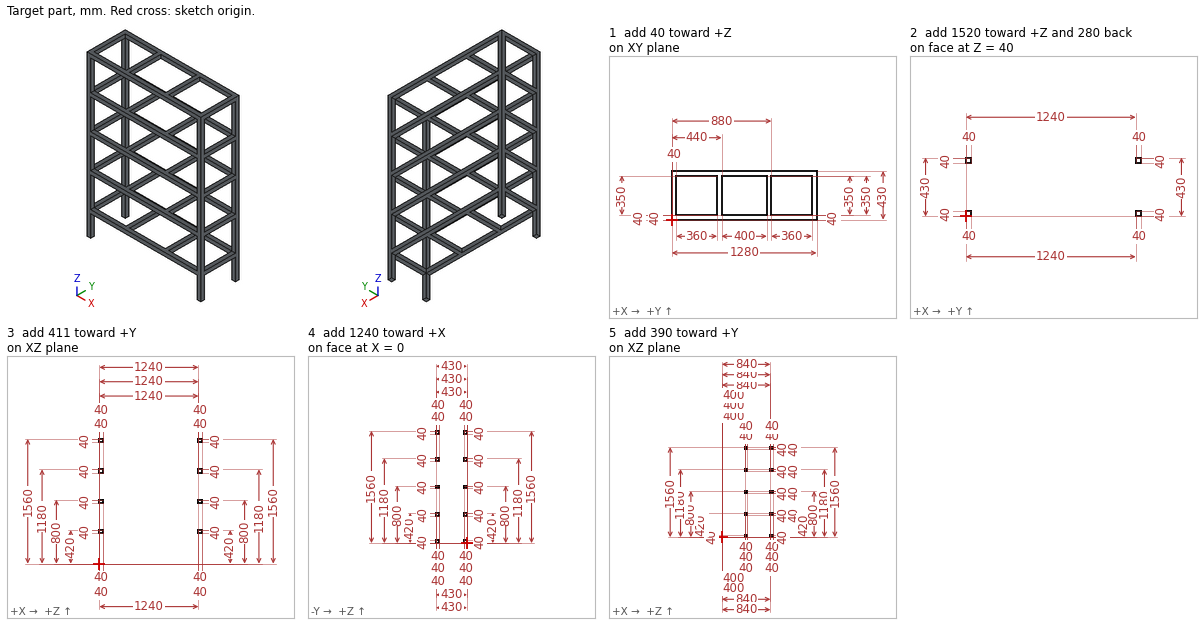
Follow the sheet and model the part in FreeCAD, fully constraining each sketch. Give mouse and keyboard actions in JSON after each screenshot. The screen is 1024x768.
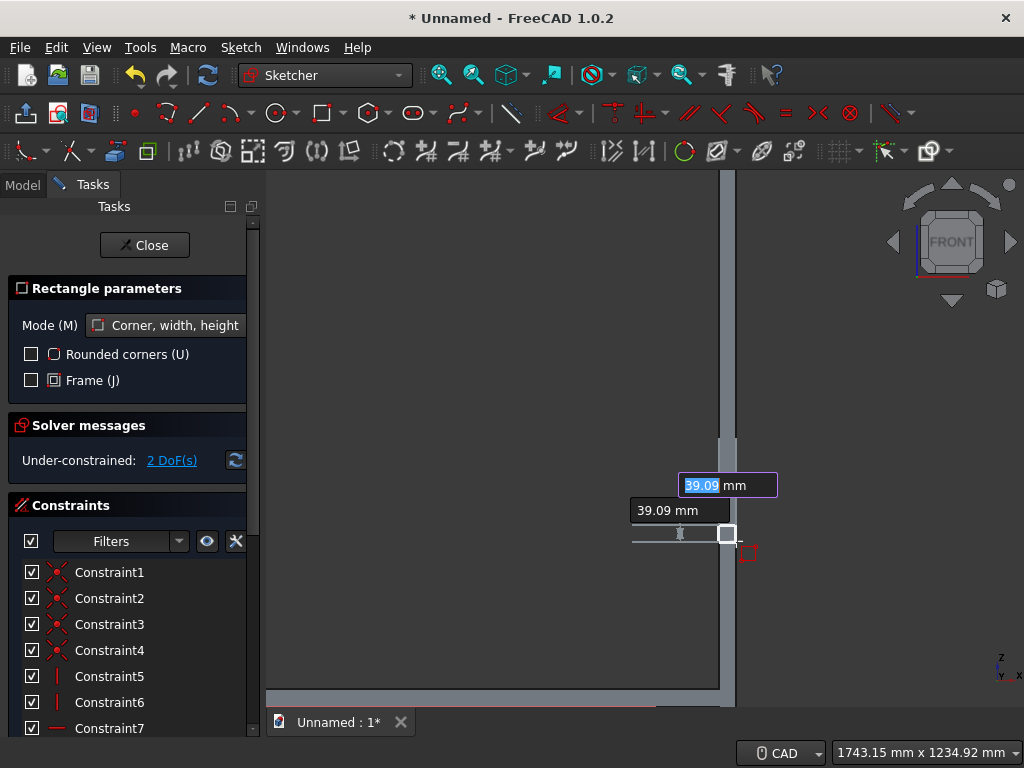
{"action": "type", "text": "40"}
{"action": "key", "text": "Tab"}
{"action": "type", "text": "40"}
{"action": "key", "text": "Return"}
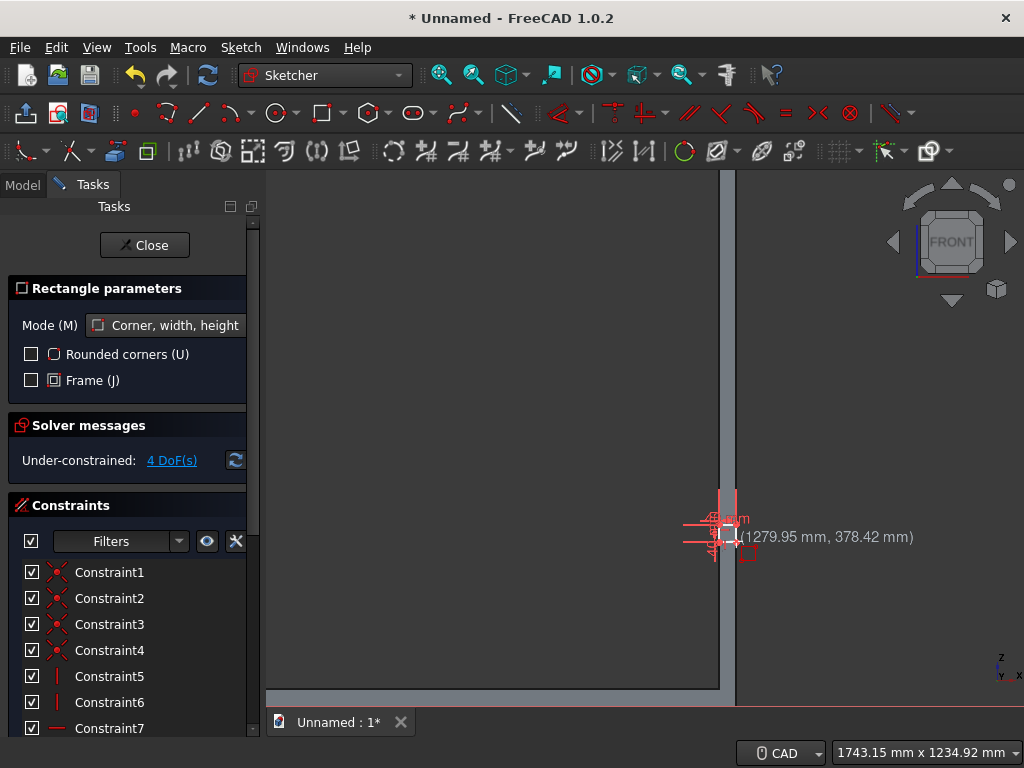
{"action": "scroll", "coordinate": [721, 525], "scroll_direction": "down", "scroll_amount": 3}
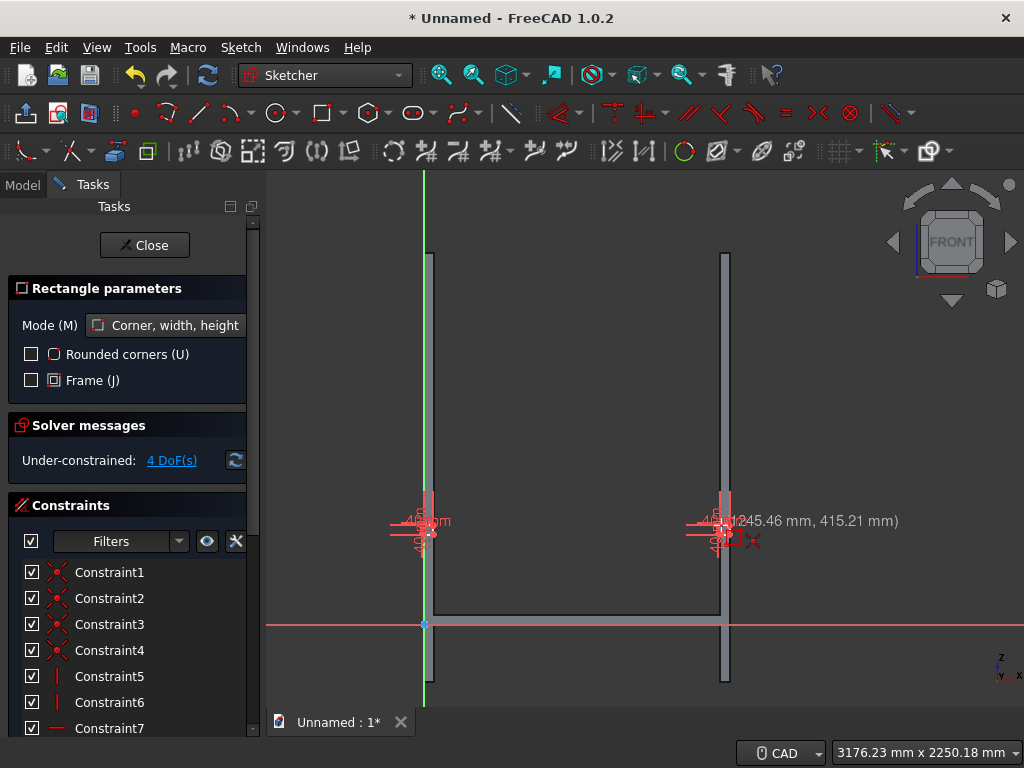
{"action": "scroll", "coordinate": [424, 434], "scroll_direction": "up", "scroll_amount": 3}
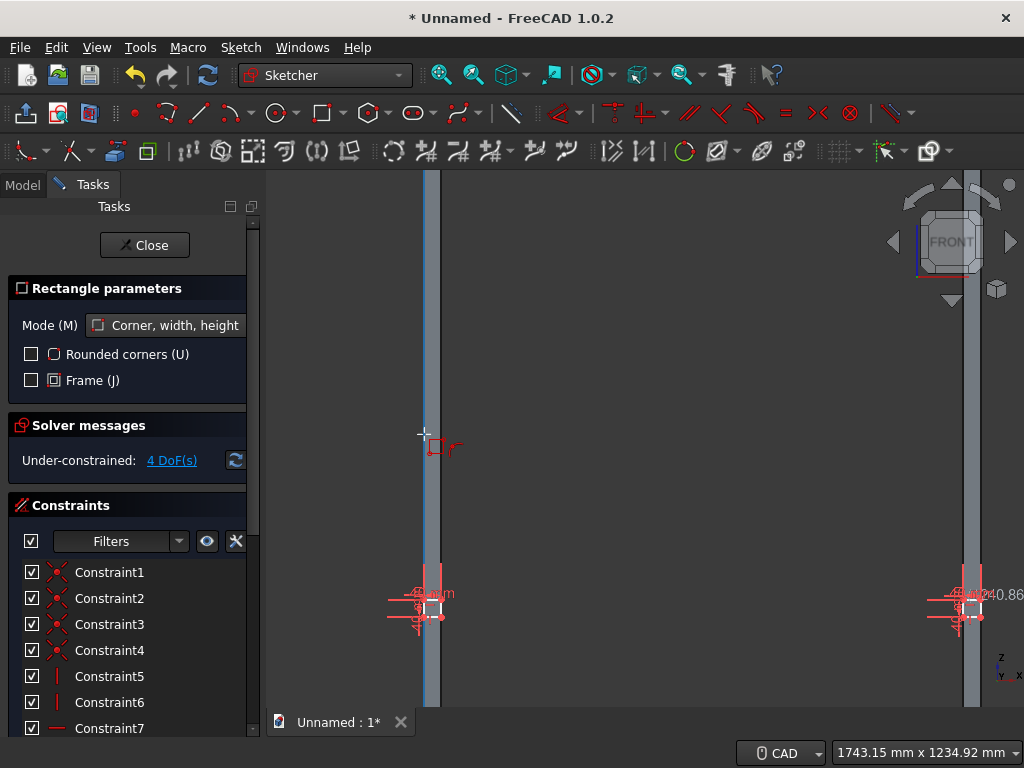
{"action": "left_click", "coordinate": [424, 434]}
{"action": "mouse_move", "coordinate": [441, 451]}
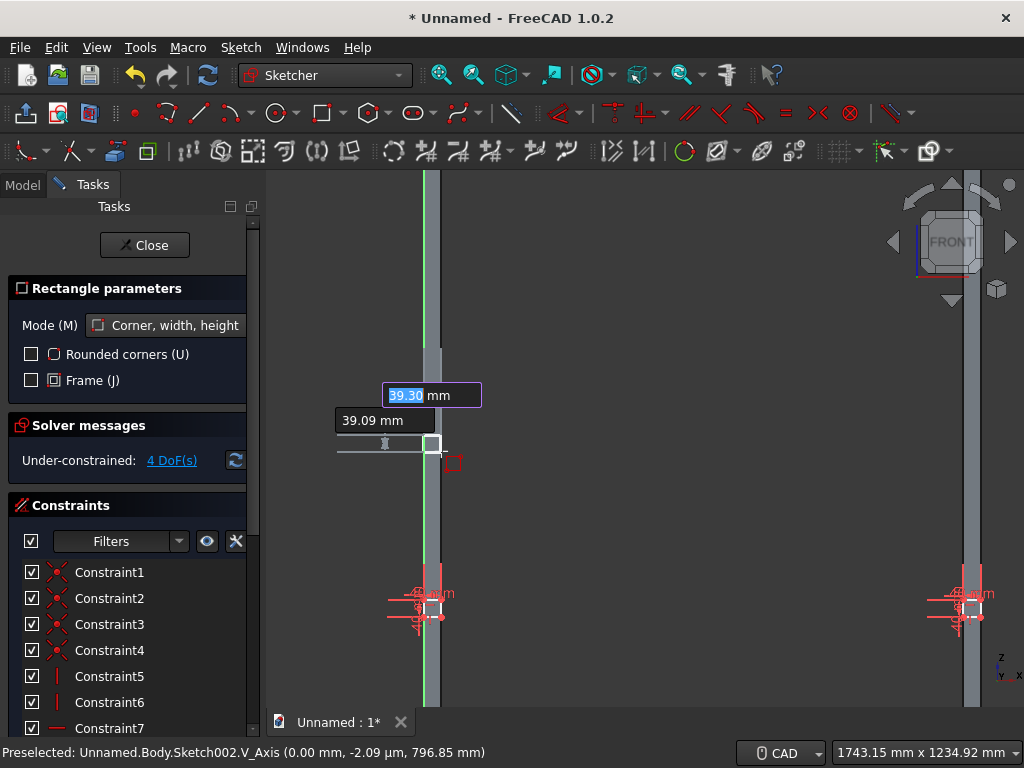
{"action": "type", "text": "40"}
{"action": "key", "text": "Tab"}
{"action": "type", "text": "40"}
{"action": "key", "text": "Return"}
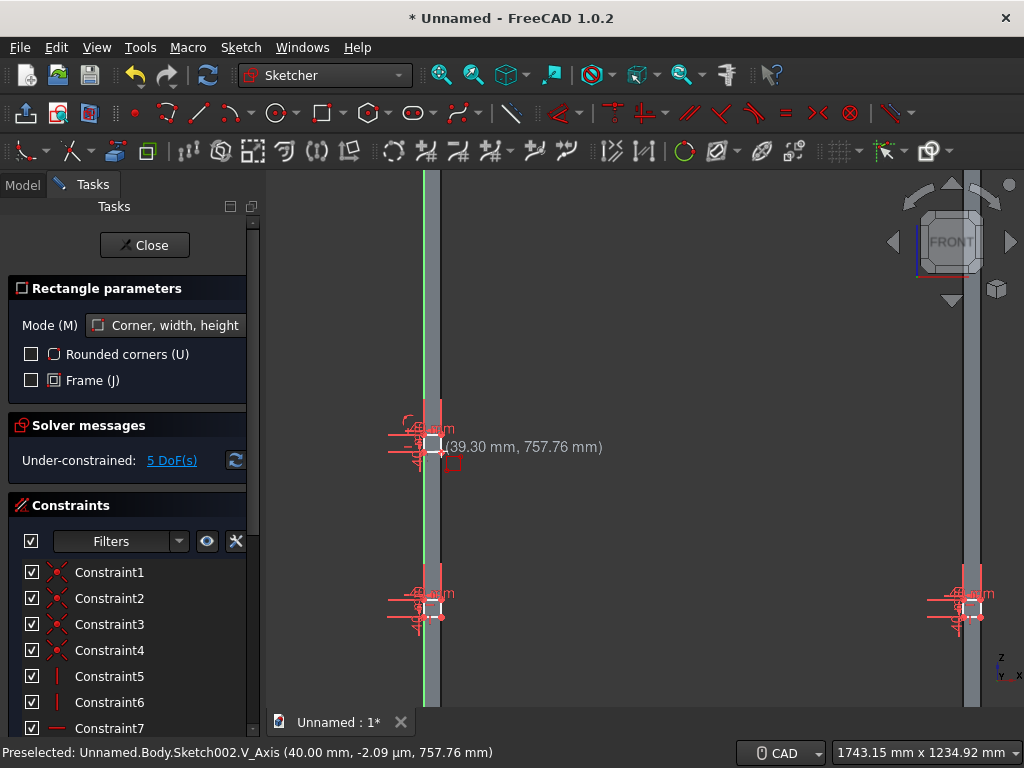
{"action": "scroll", "coordinate": [424, 434], "scroll_direction": "down", "scroll_amount": 3}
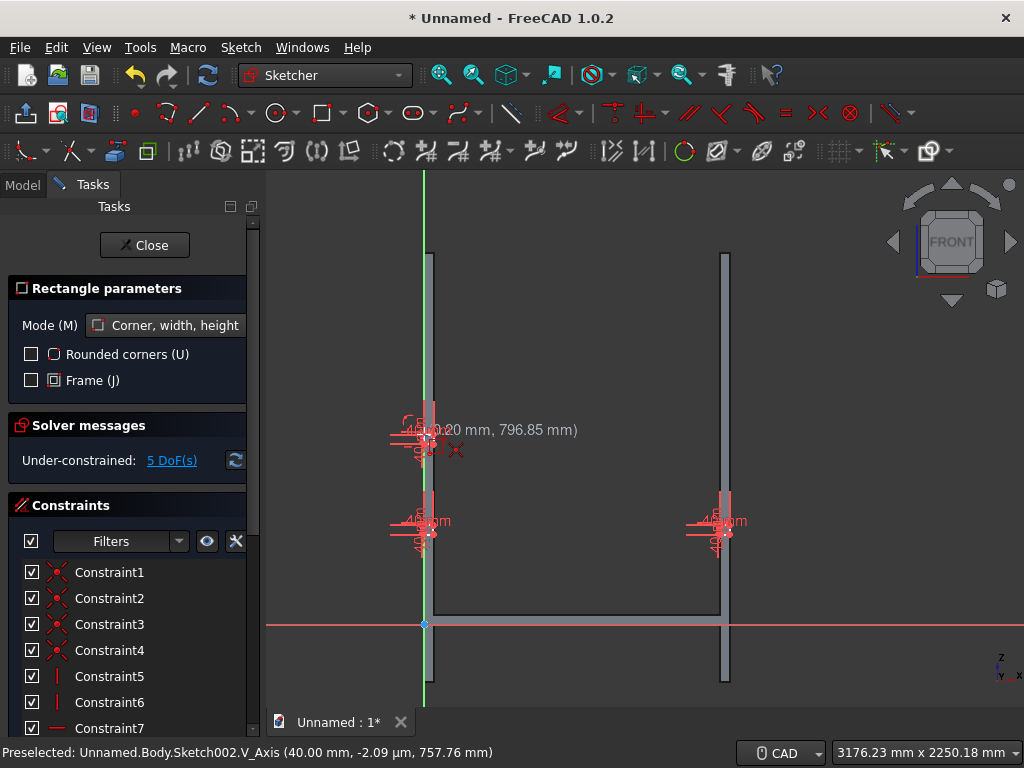
{"action": "scroll", "coordinate": [720, 434], "scroll_direction": "up", "scroll_amount": 3}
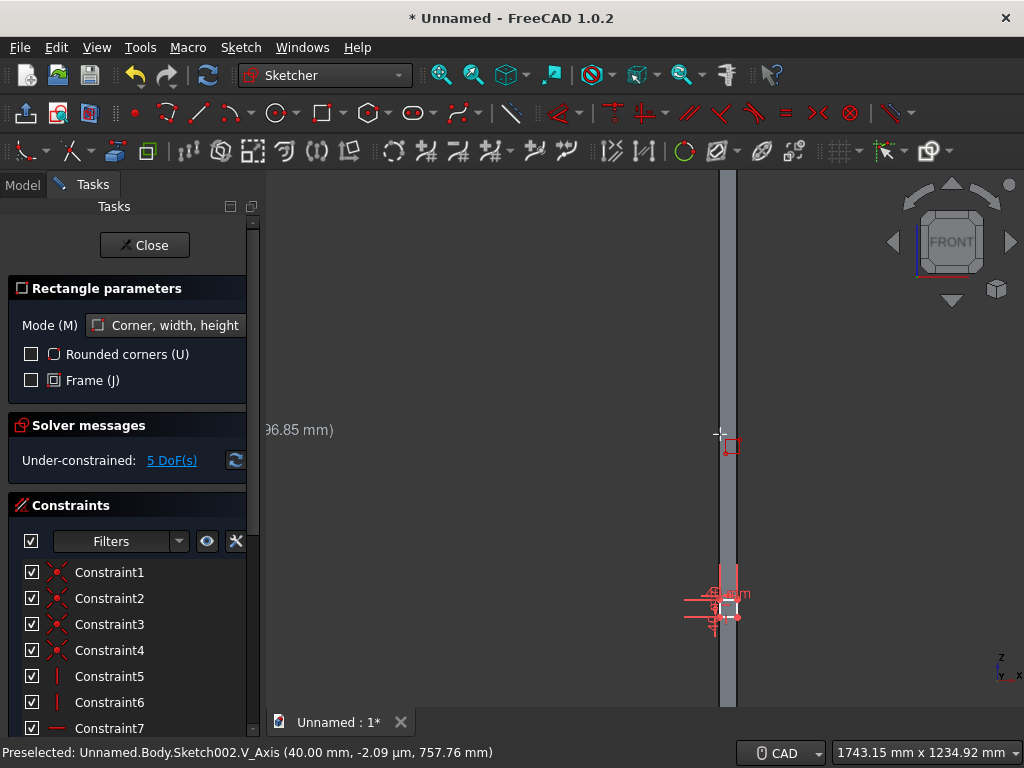
{"action": "left_click", "coordinate": [719, 434]}
{"action": "mouse_move", "coordinate": [737, 451]}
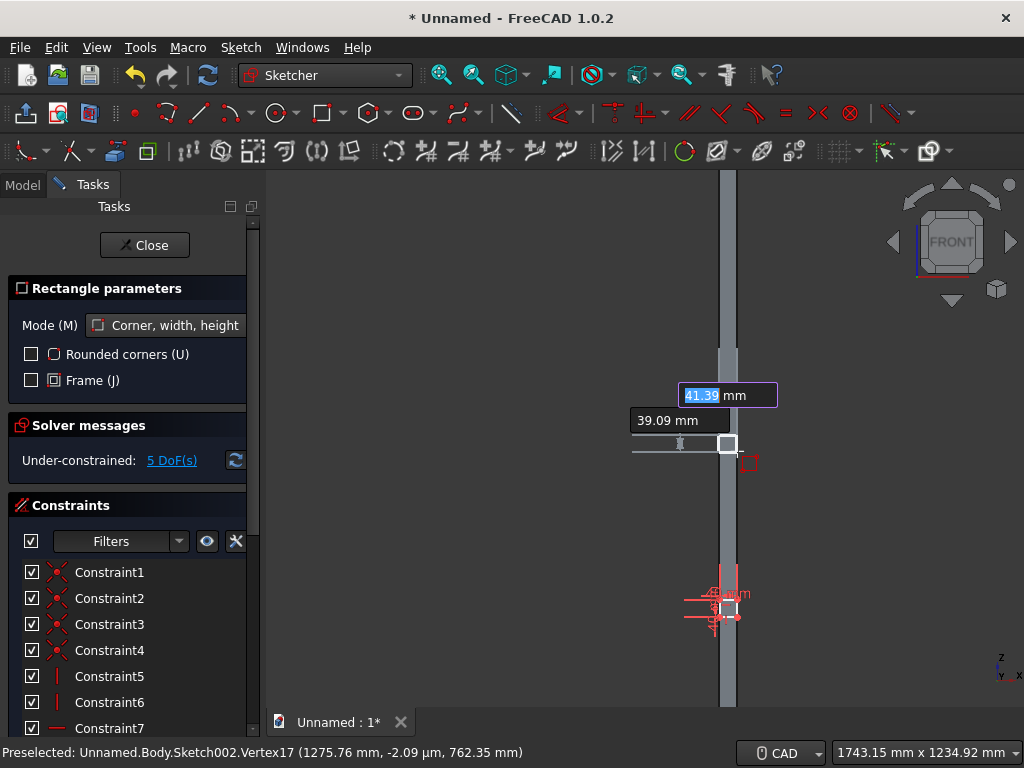
{"action": "type", "text": "40"}
{"action": "key", "text": "Tab"}
{"action": "type", "text": "40"}
{"action": "key", "text": "Return"}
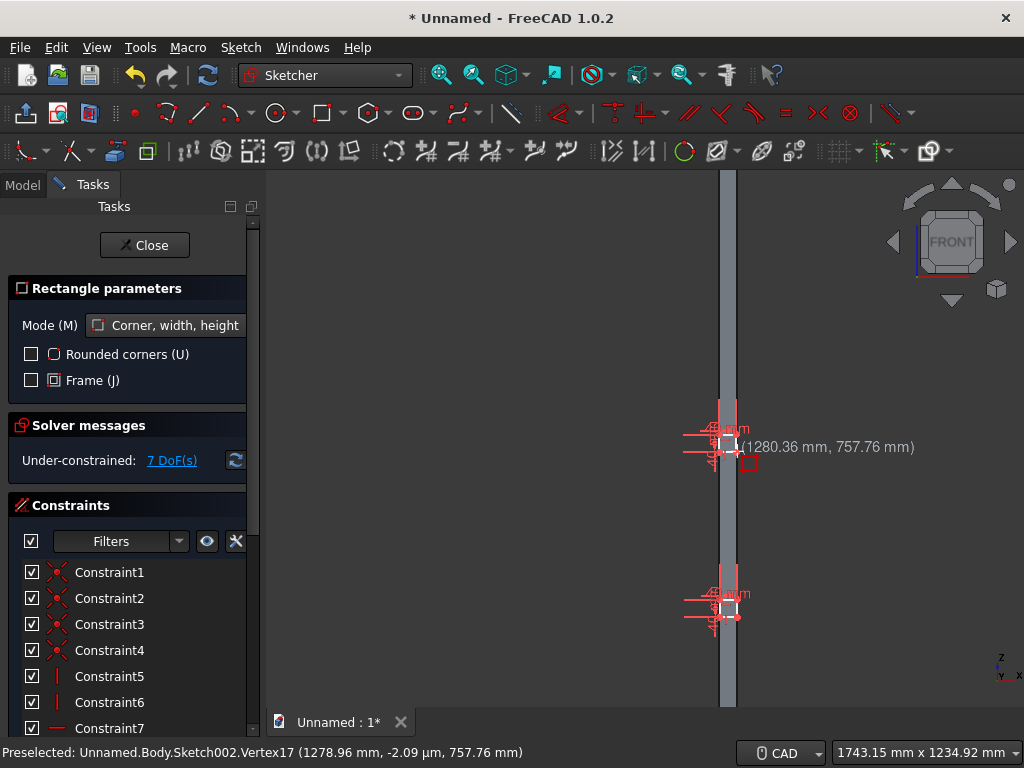
{"action": "scroll", "coordinate": [720, 434], "scroll_direction": "down", "scroll_amount": 3}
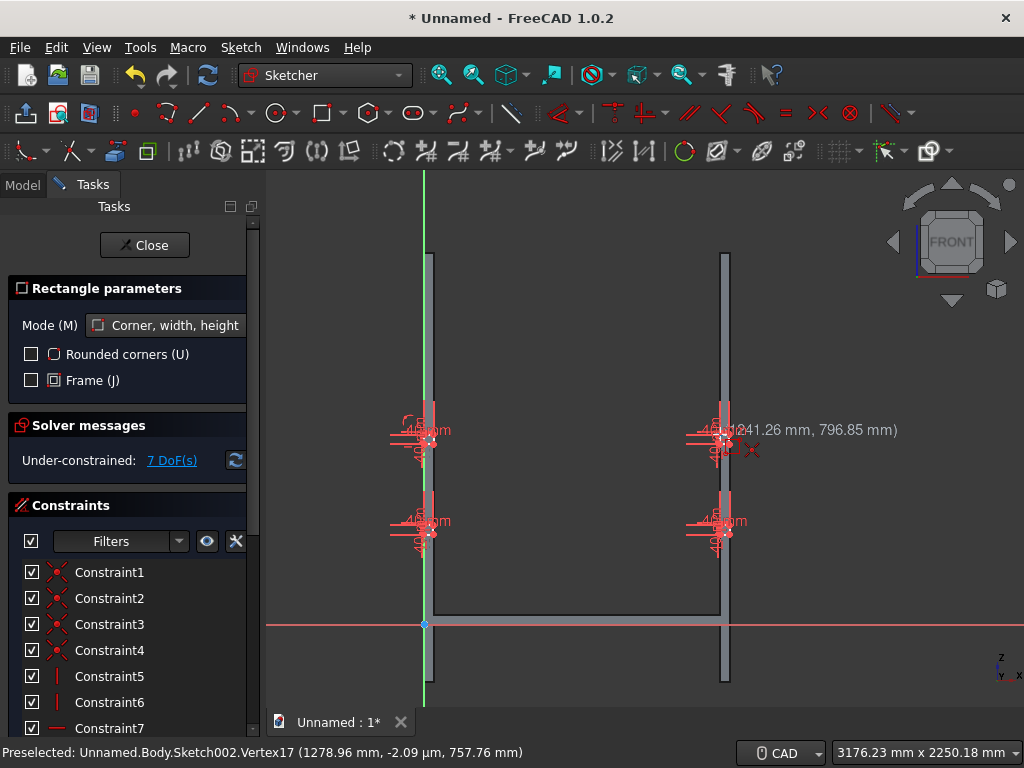
{"action": "scroll", "coordinate": [424, 343], "scroll_direction": "up", "scroll_amount": 3}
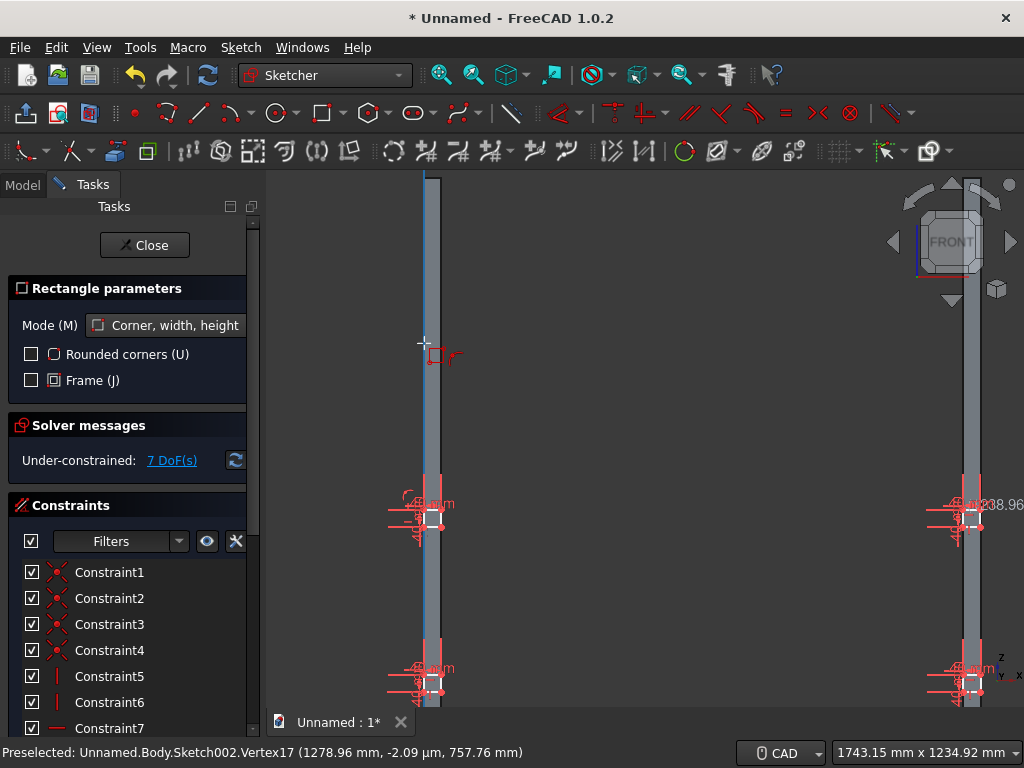
{"action": "left_click", "coordinate": [424, 343]}
{"action": "mouse_move", "coordinate": [441, 361]}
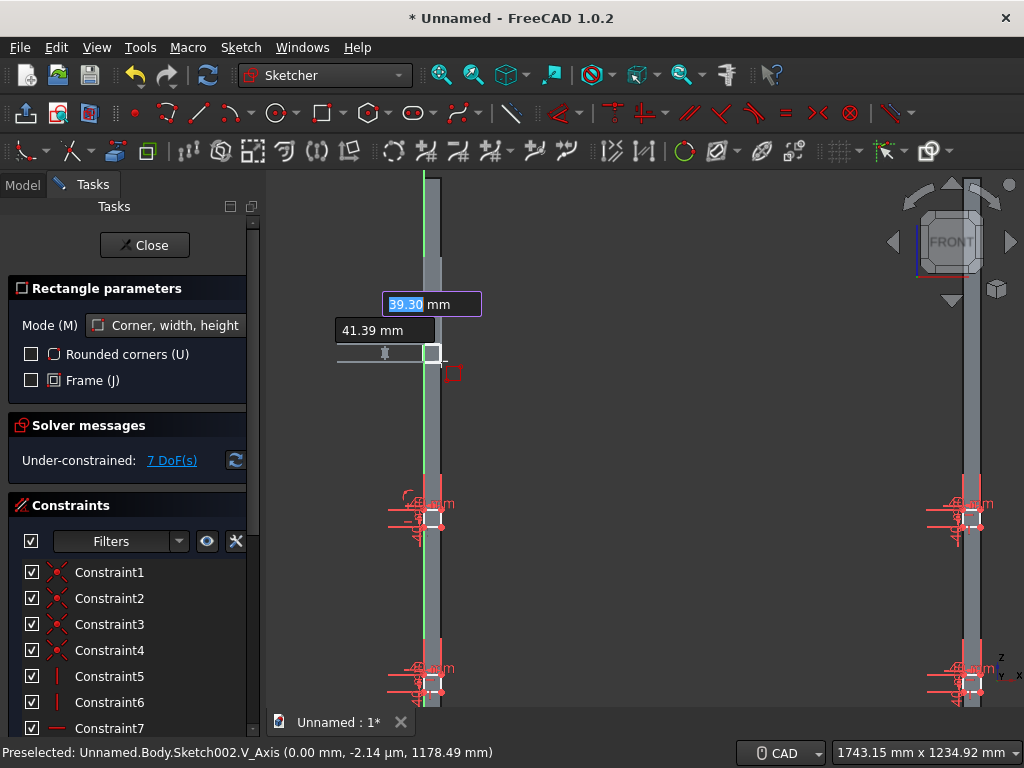
{"action": "type", "text": "40"}
{"action": "key", "text": "Tab"}
{"action": "type", "text": "40"}
{"action": "key", "text": "Return"}